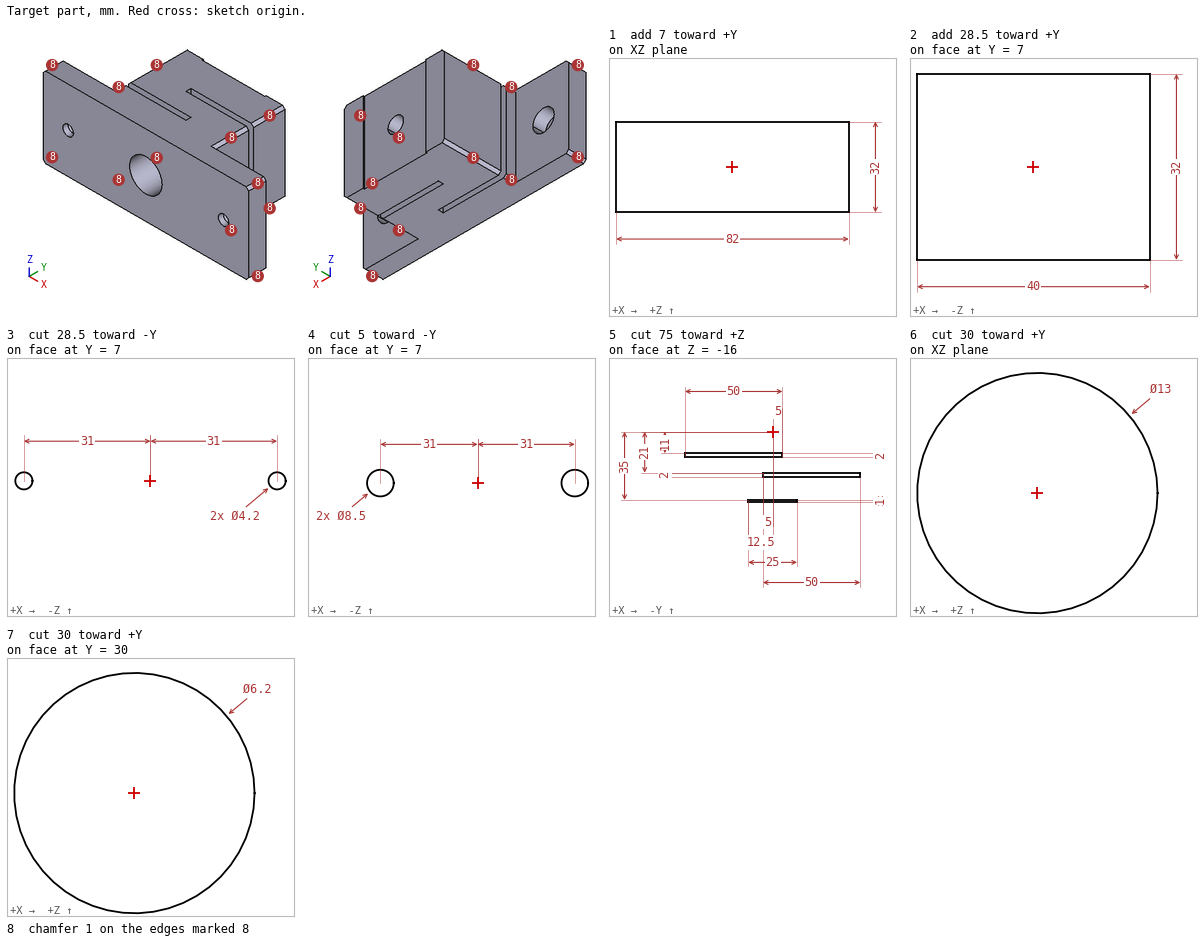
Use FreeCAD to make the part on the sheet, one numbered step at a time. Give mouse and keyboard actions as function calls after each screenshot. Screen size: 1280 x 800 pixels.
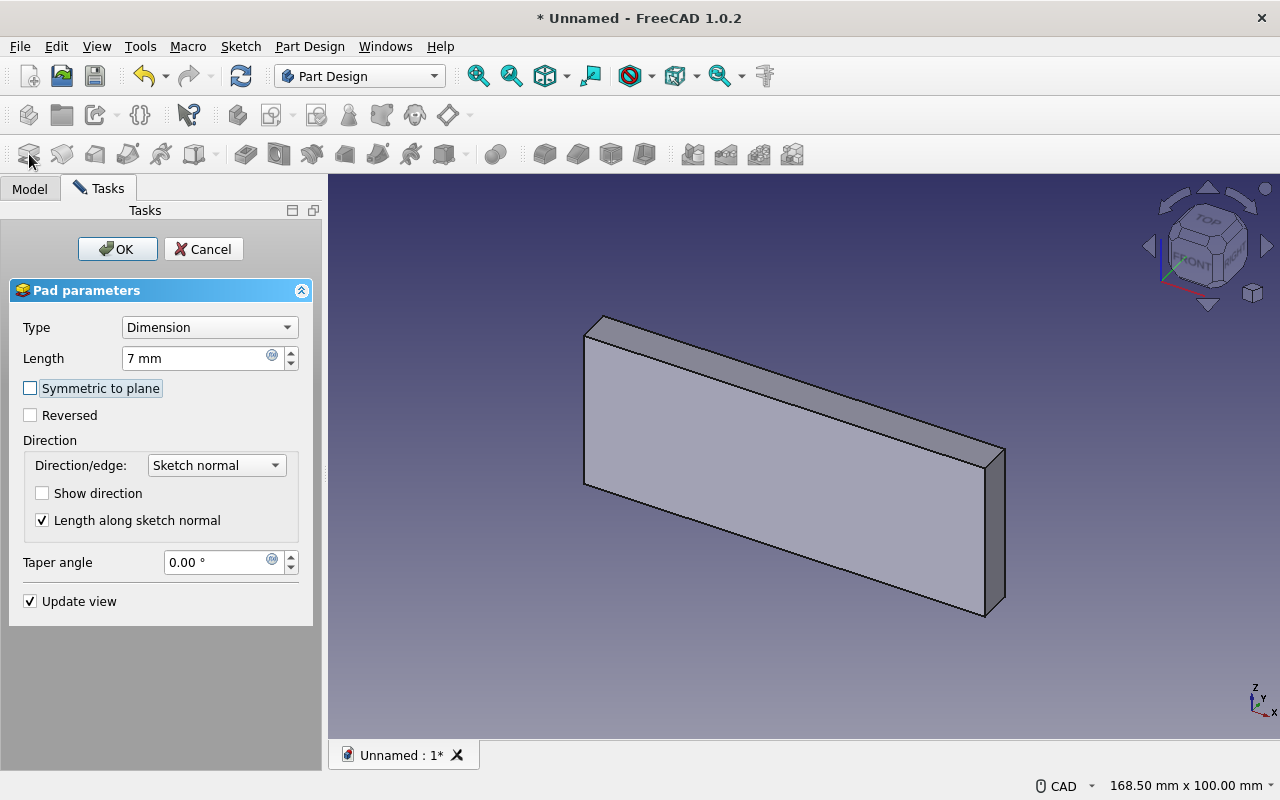
click(31, 415)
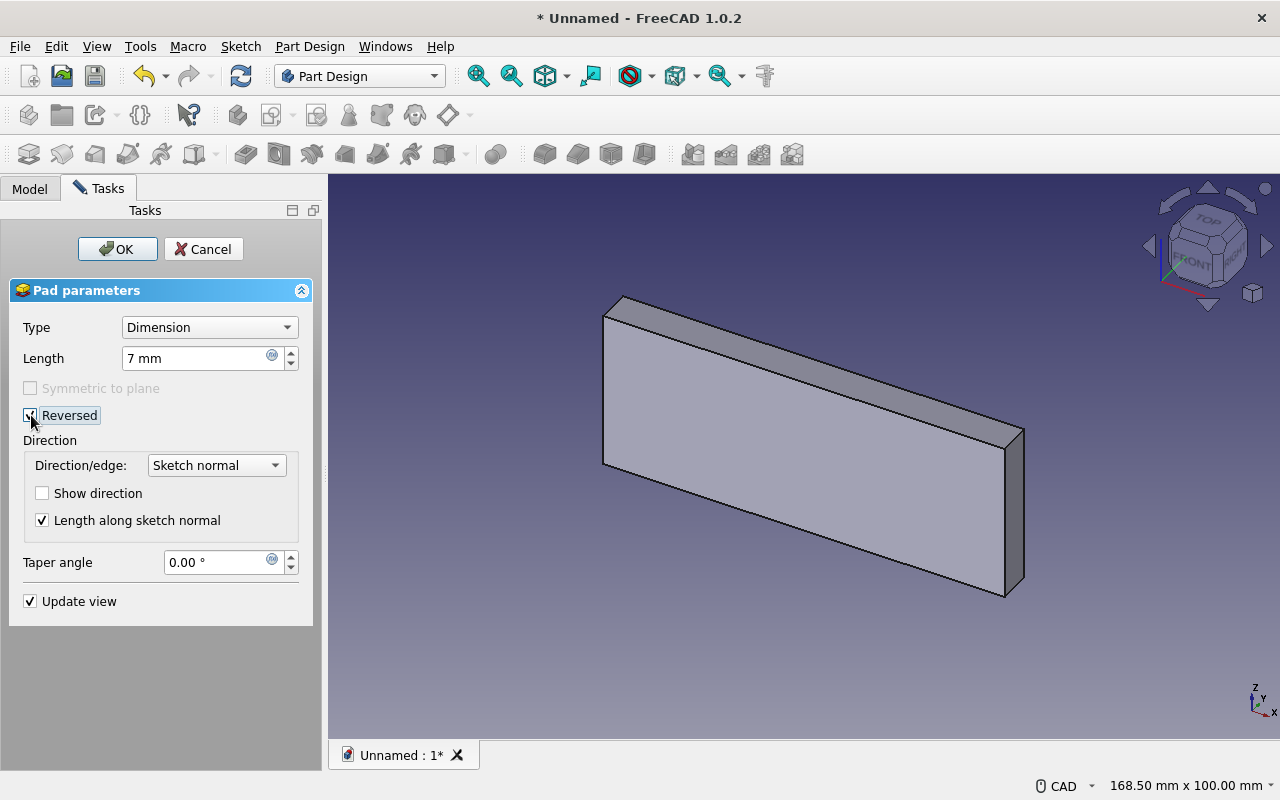
click(118, 249)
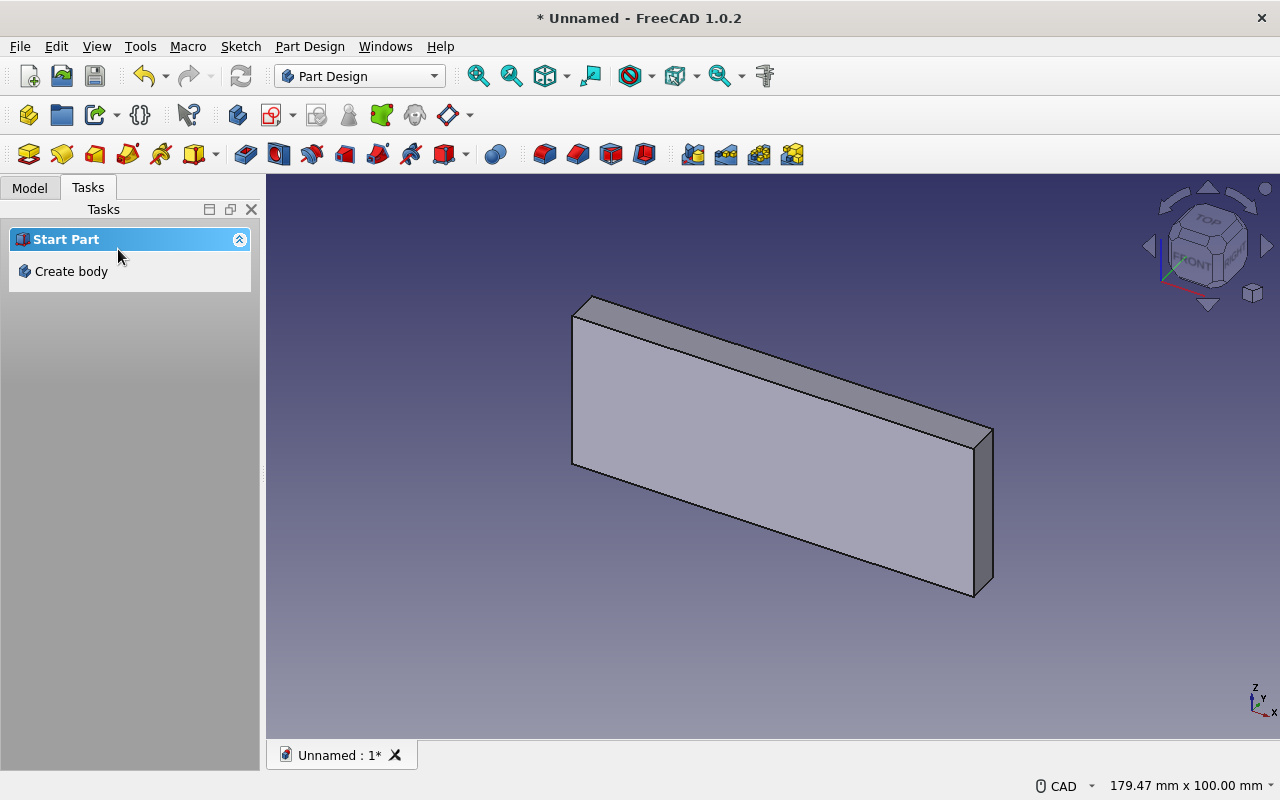
key(4)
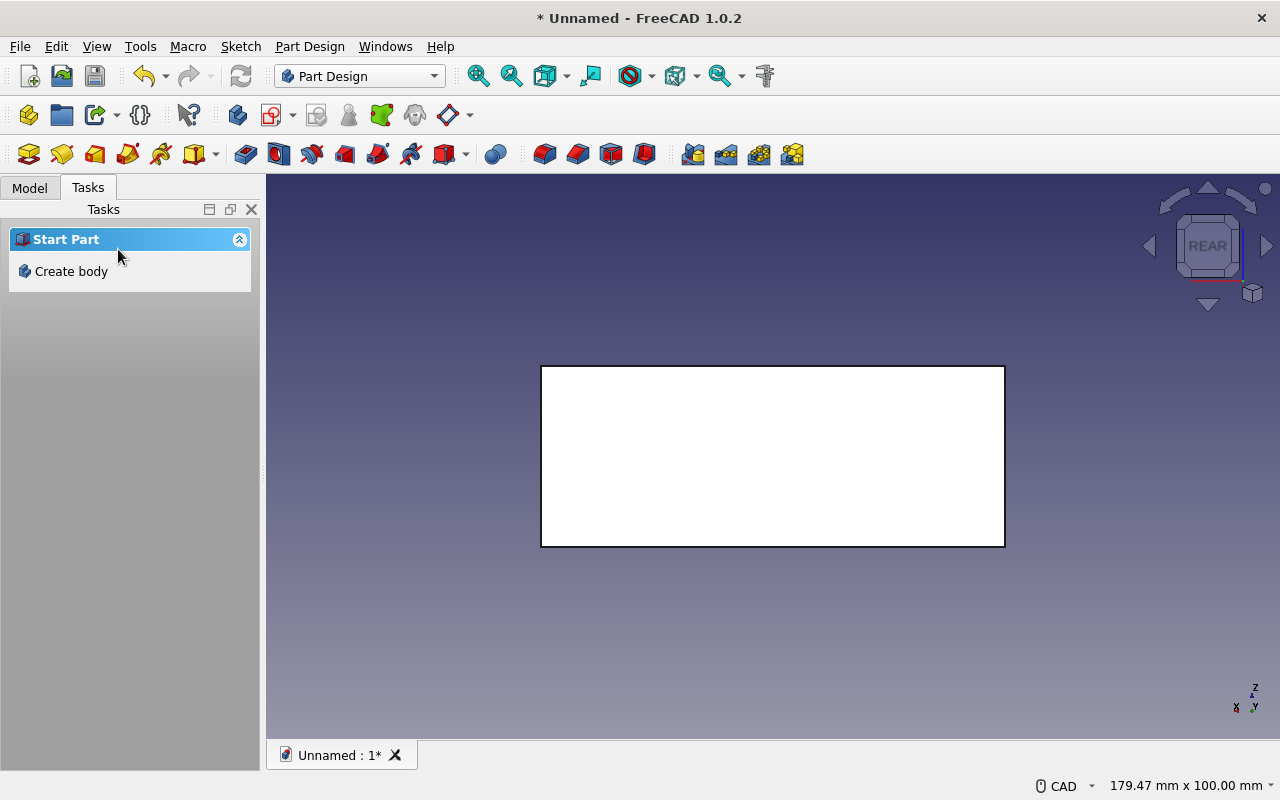
click(641, 455)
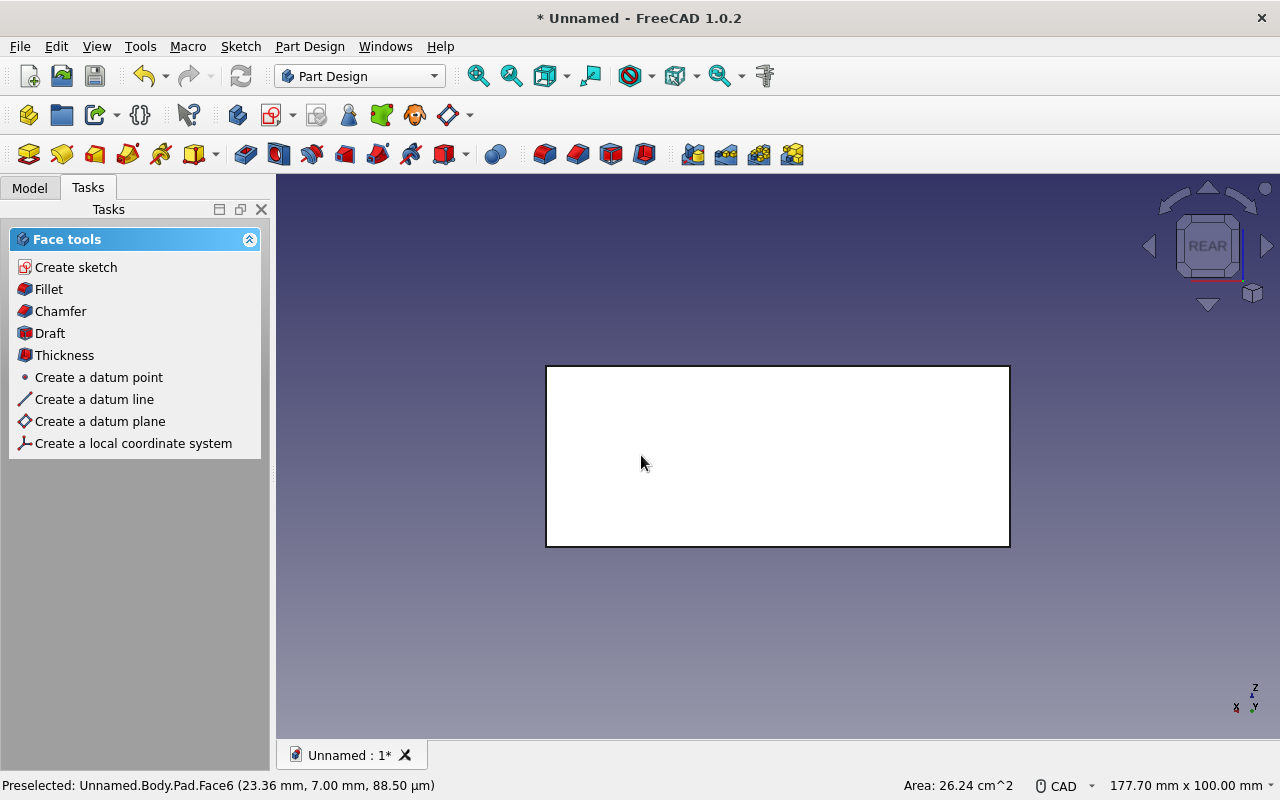
click(270, 116)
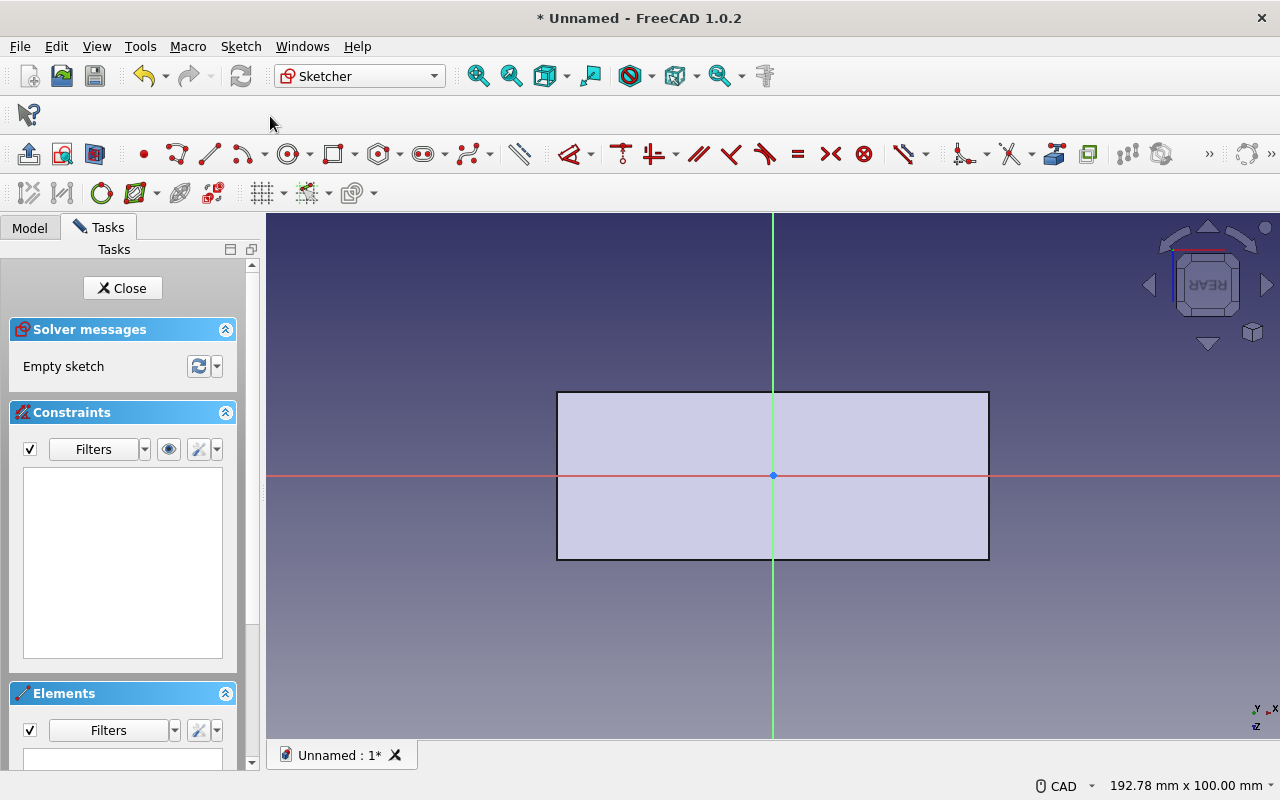
scroll(856, 476, up, 3)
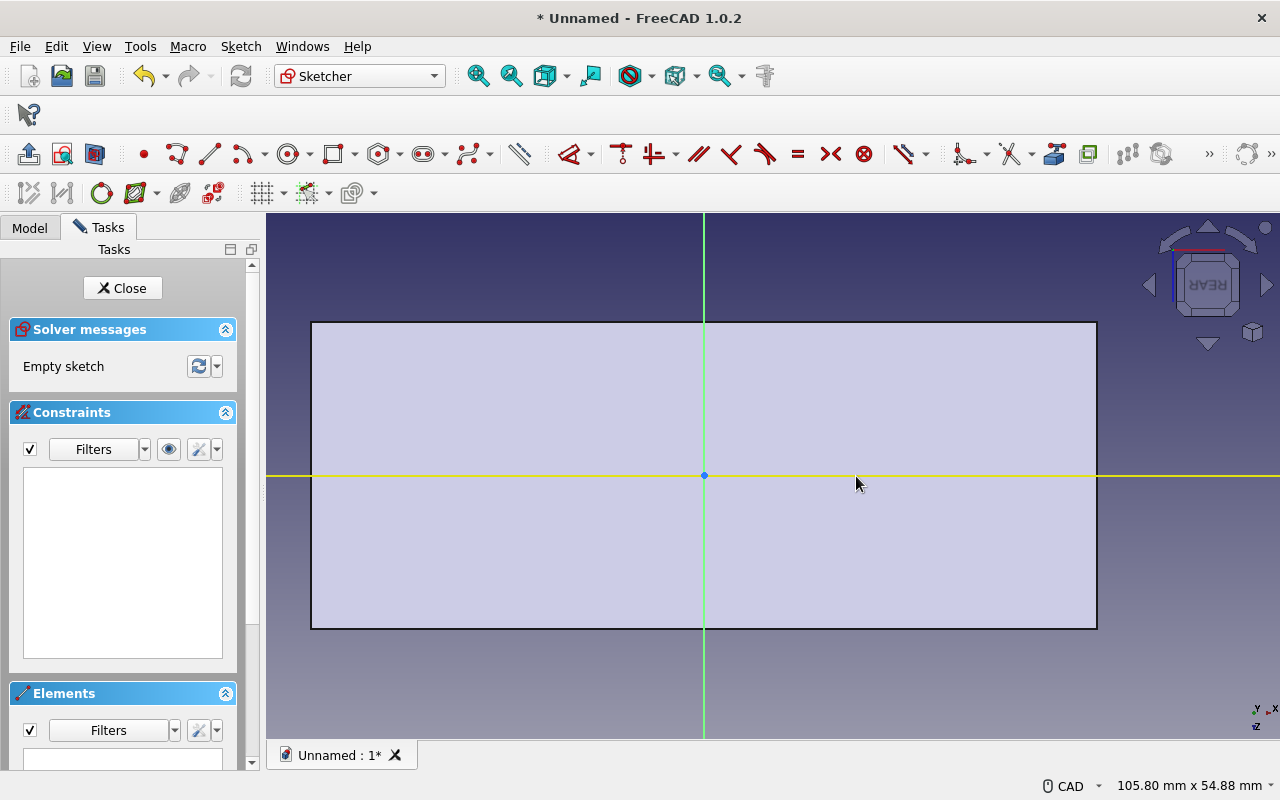
click(354, 154)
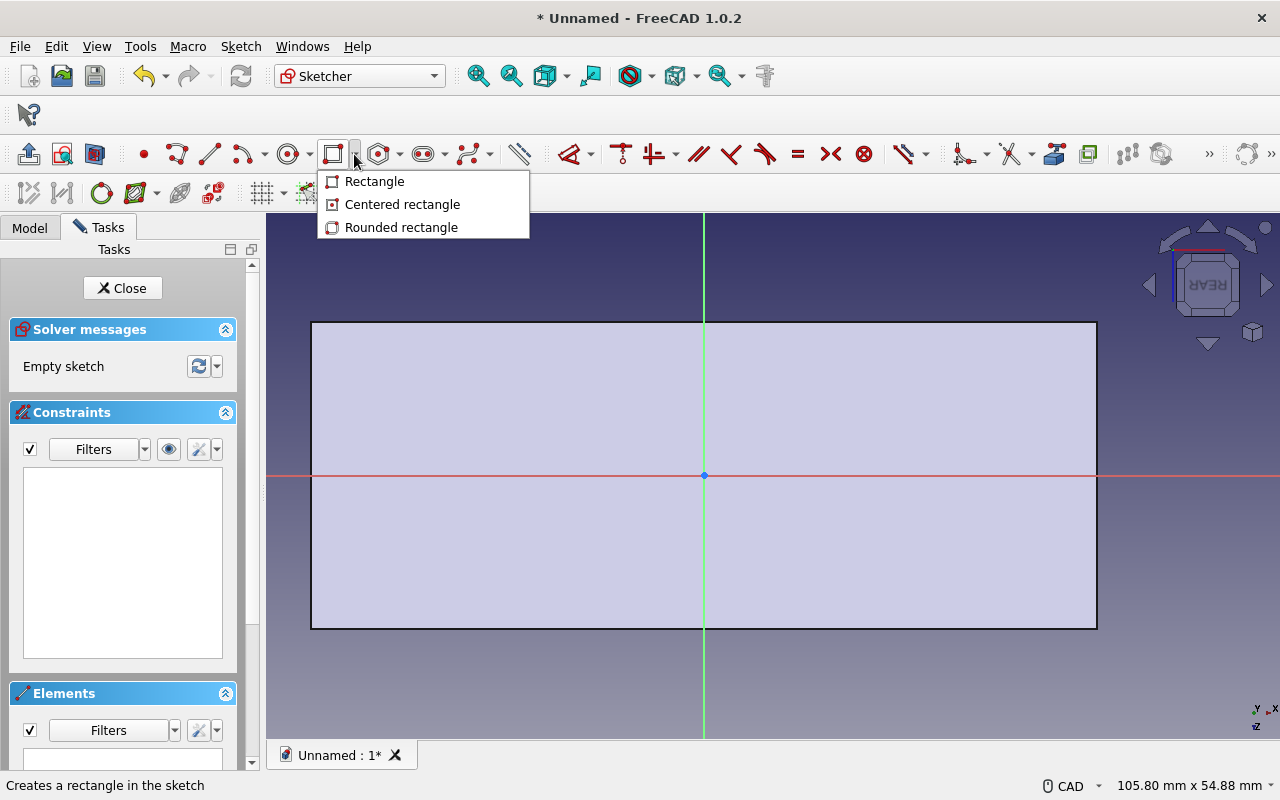
click(424, 204)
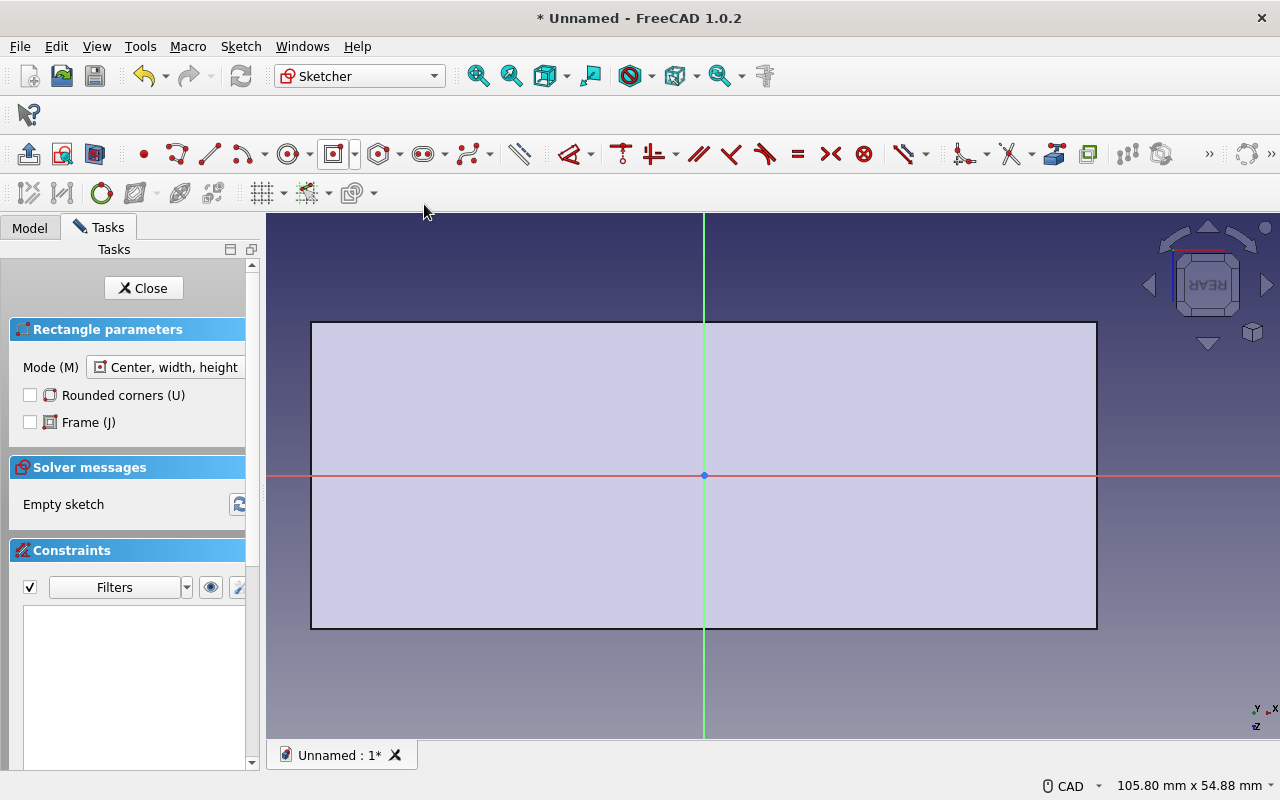
click(704, 476)
move(896, 322)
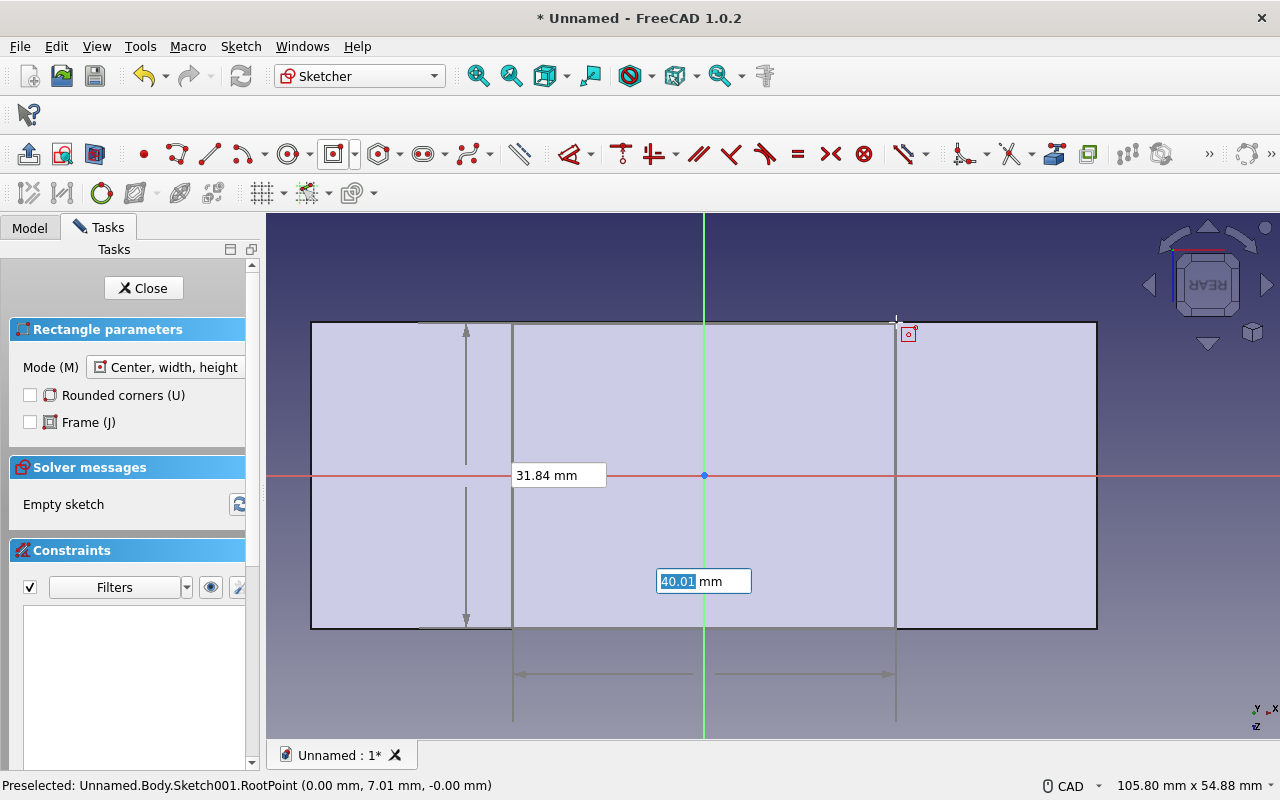
text(40)
key(Tab)
text(32)
key(Return)
key(Escape)